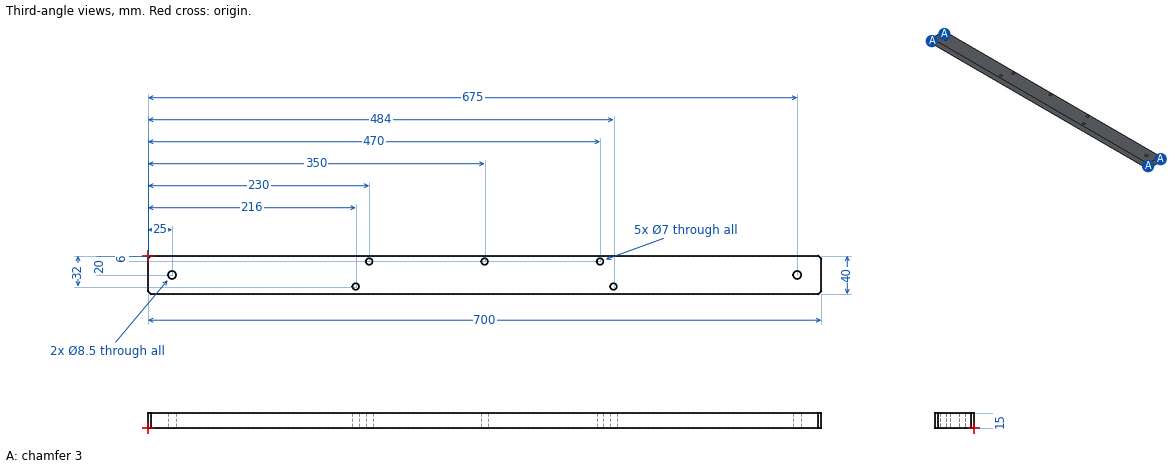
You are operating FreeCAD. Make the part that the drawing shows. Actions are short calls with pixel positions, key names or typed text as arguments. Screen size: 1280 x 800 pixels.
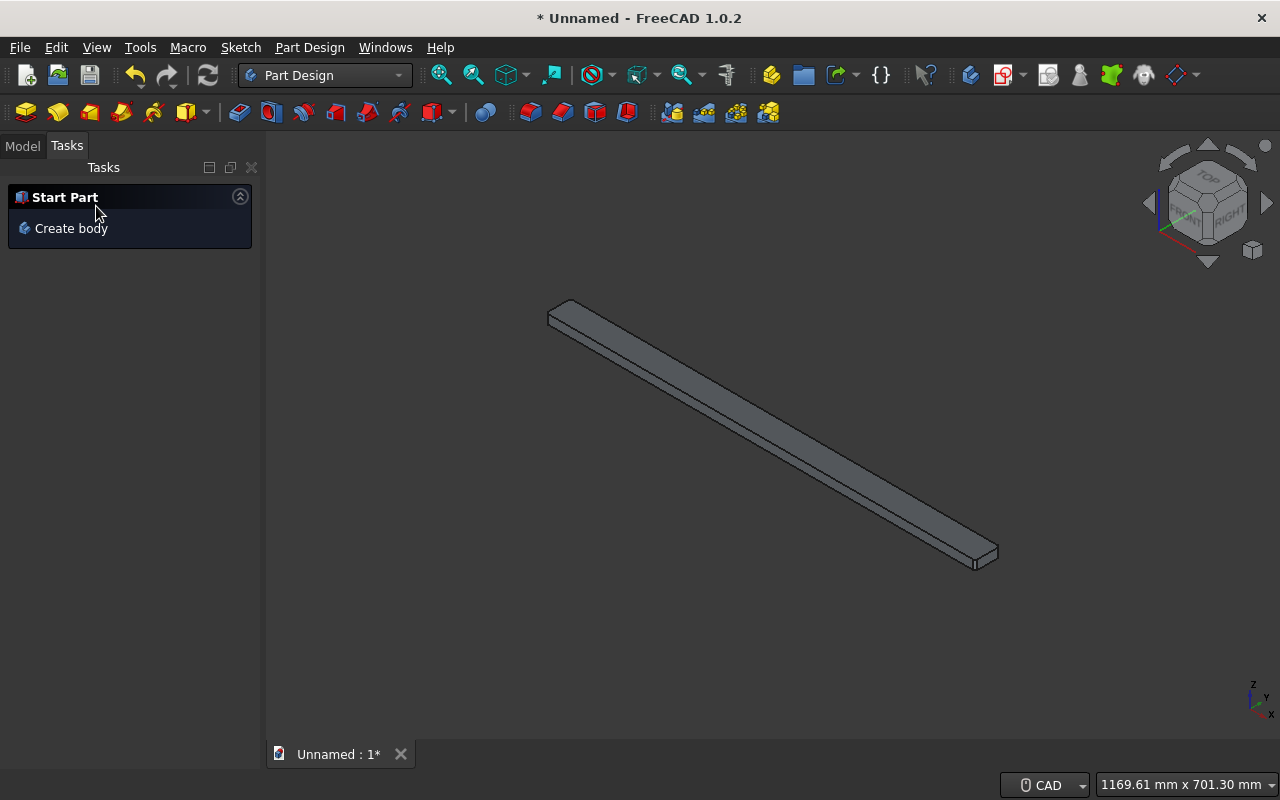
click(442, 76)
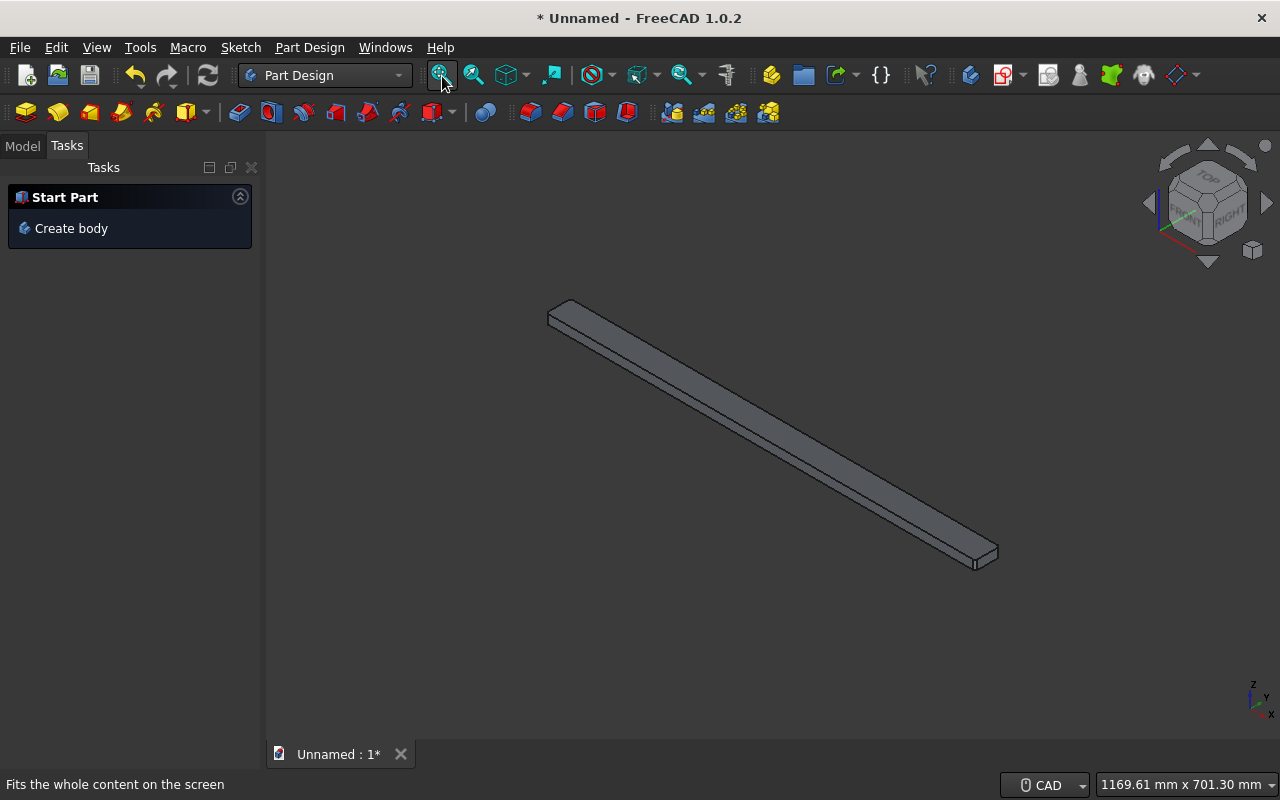
click(957, 535)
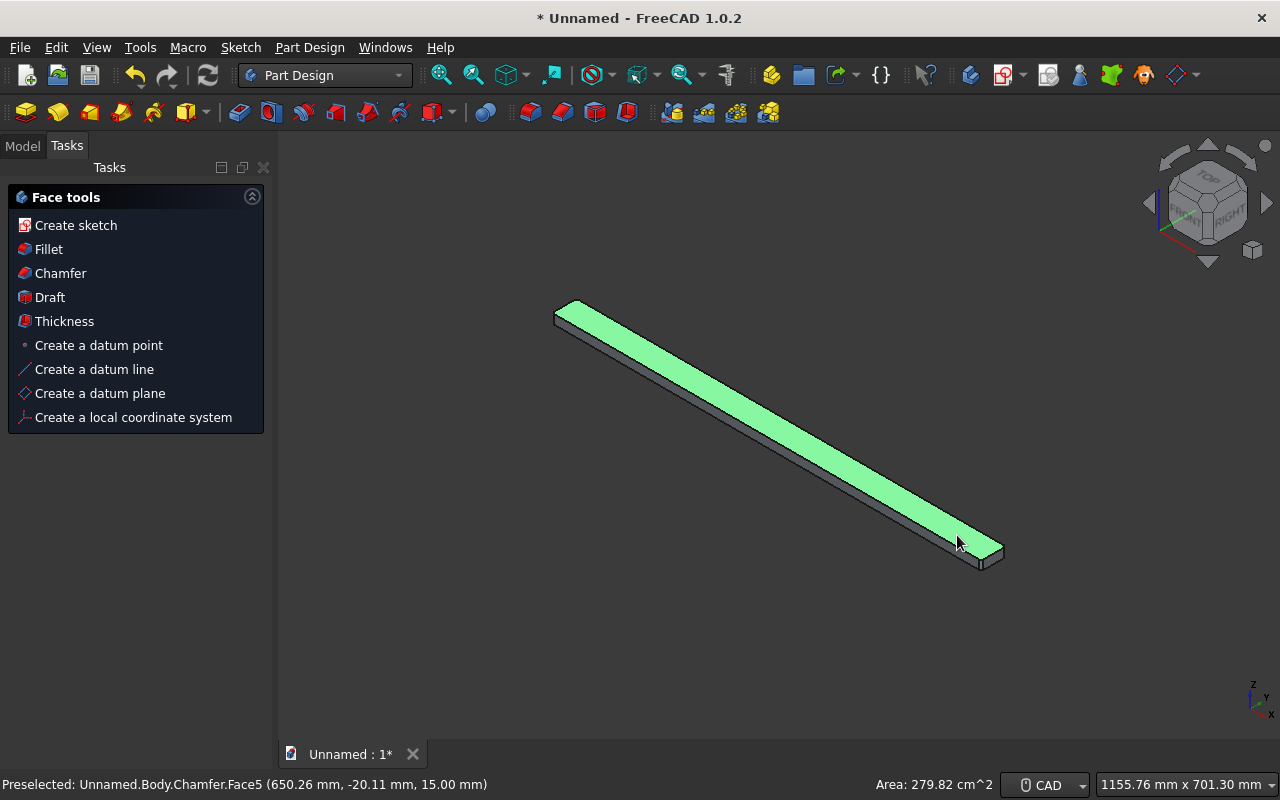
click(1004, 76)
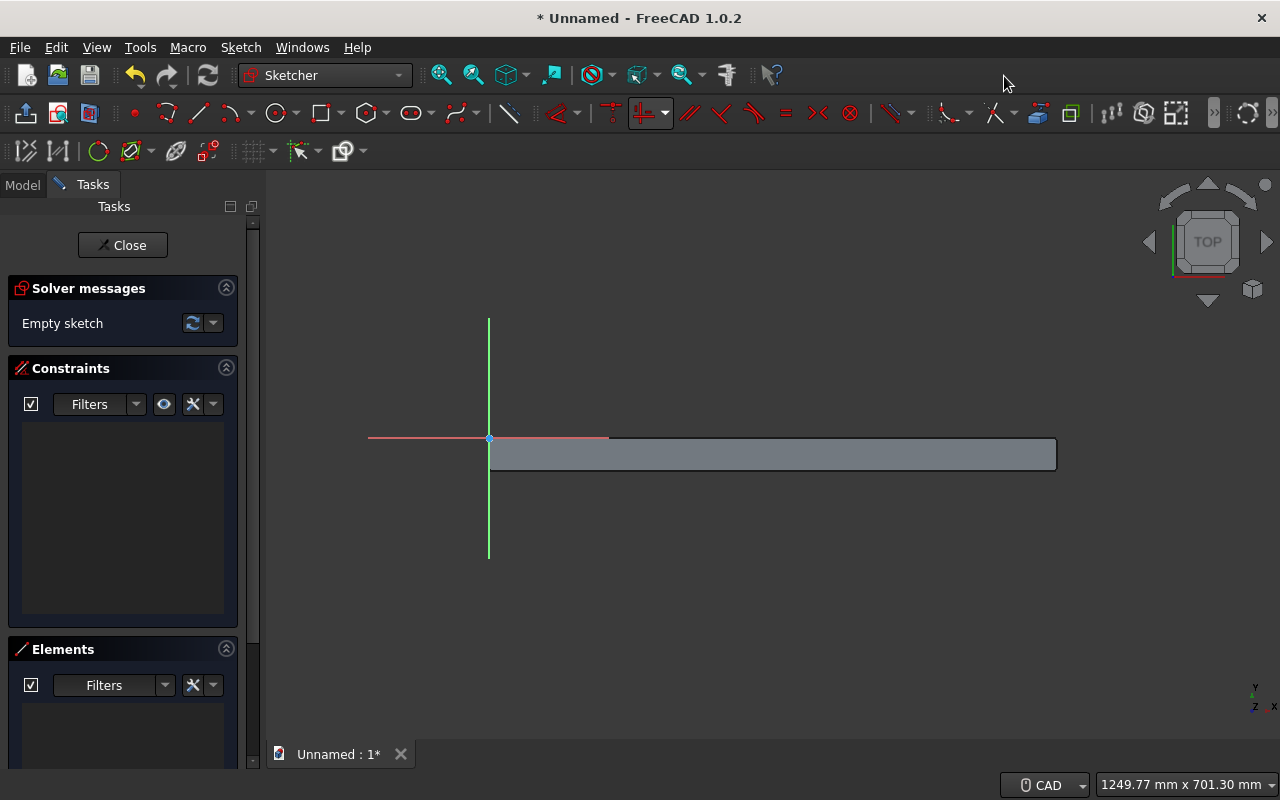
click(276, 114)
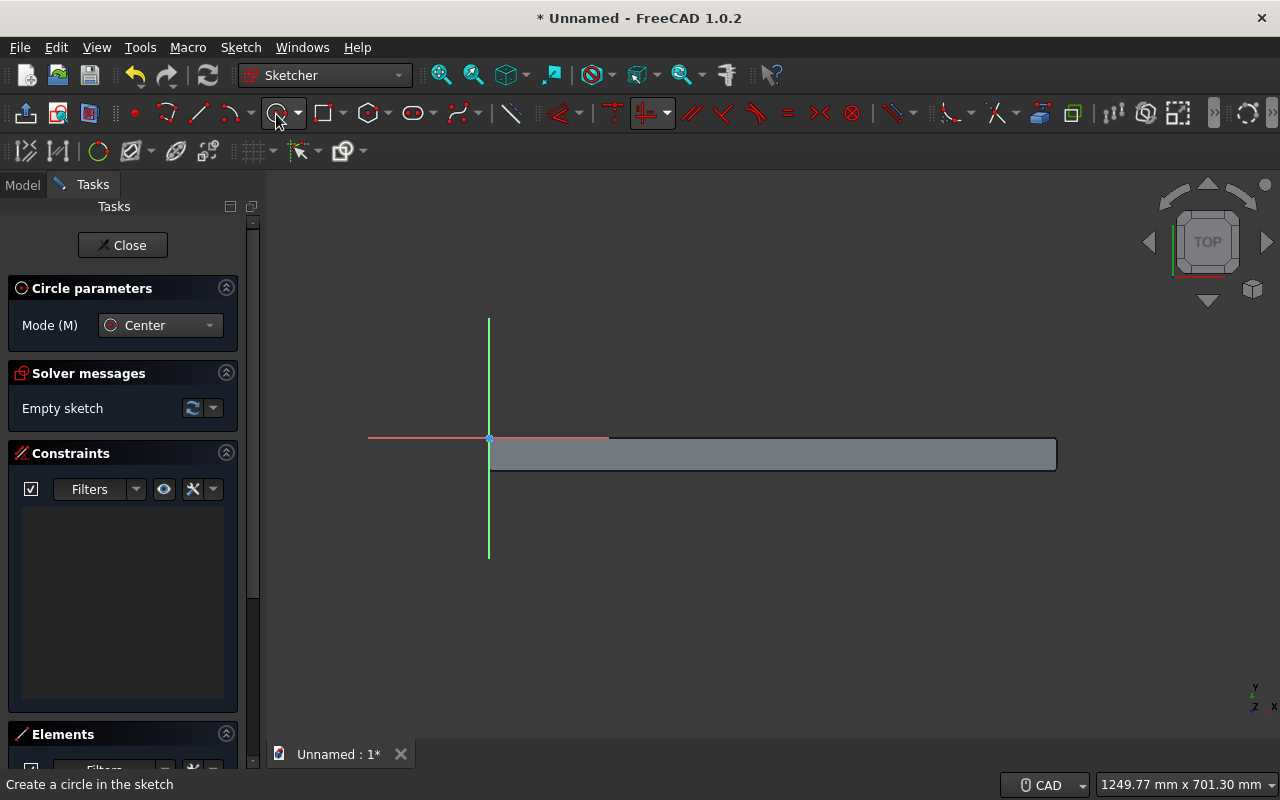
scroll(509, 454, up, 10)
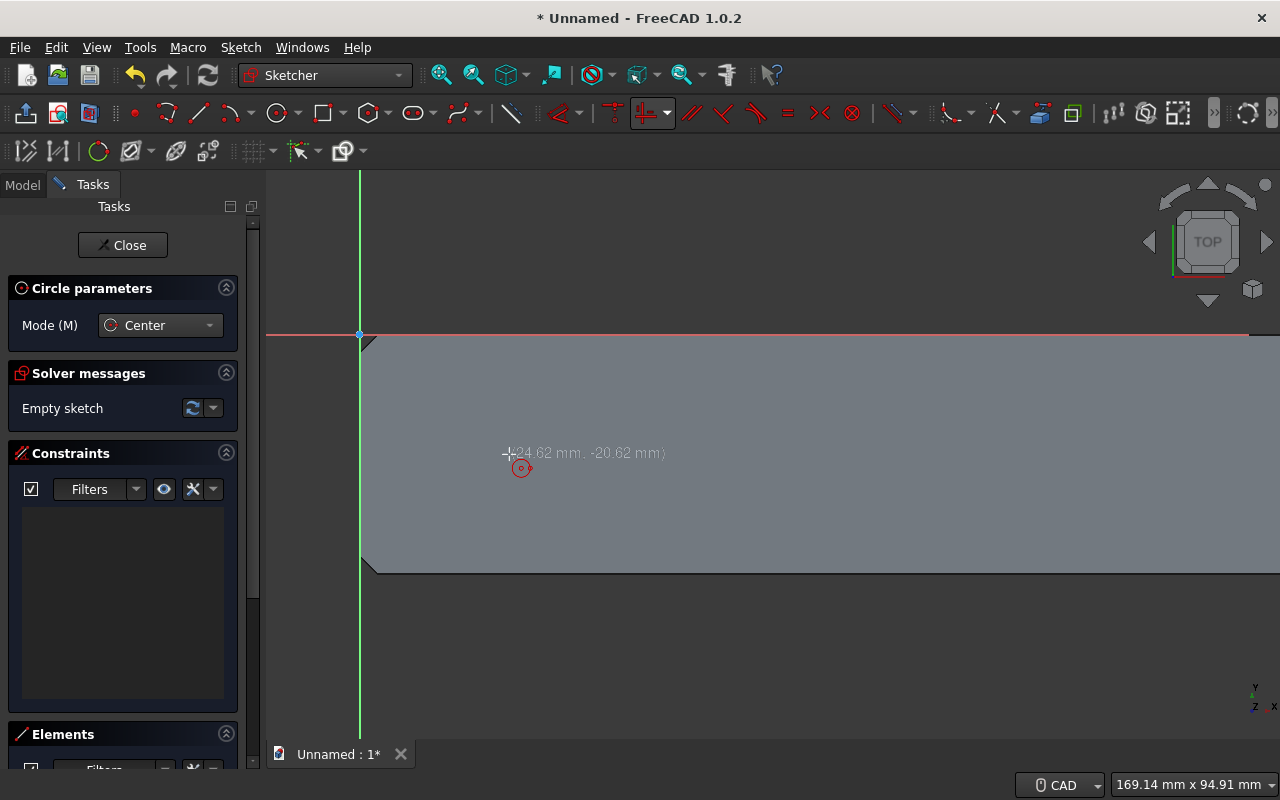
scroll(440, 462, down, 10)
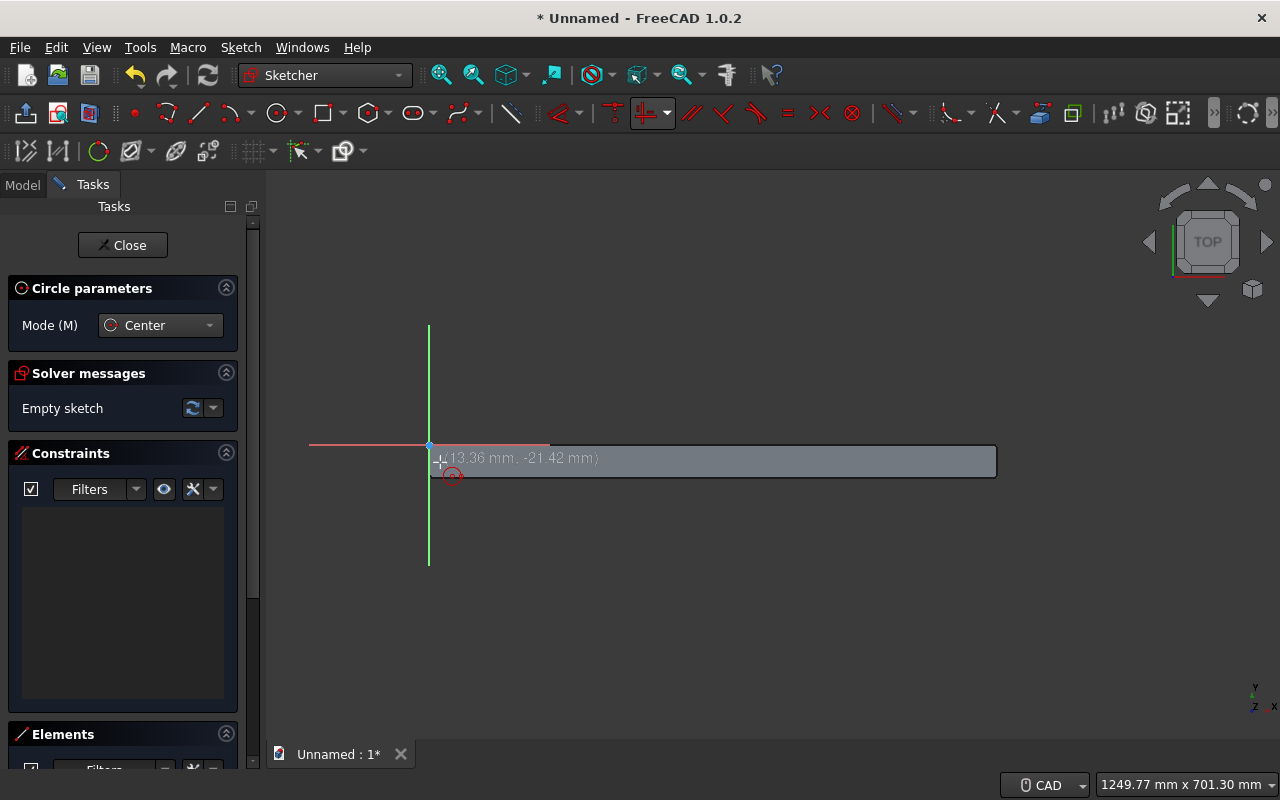
click(450, 461)
move(452, 464)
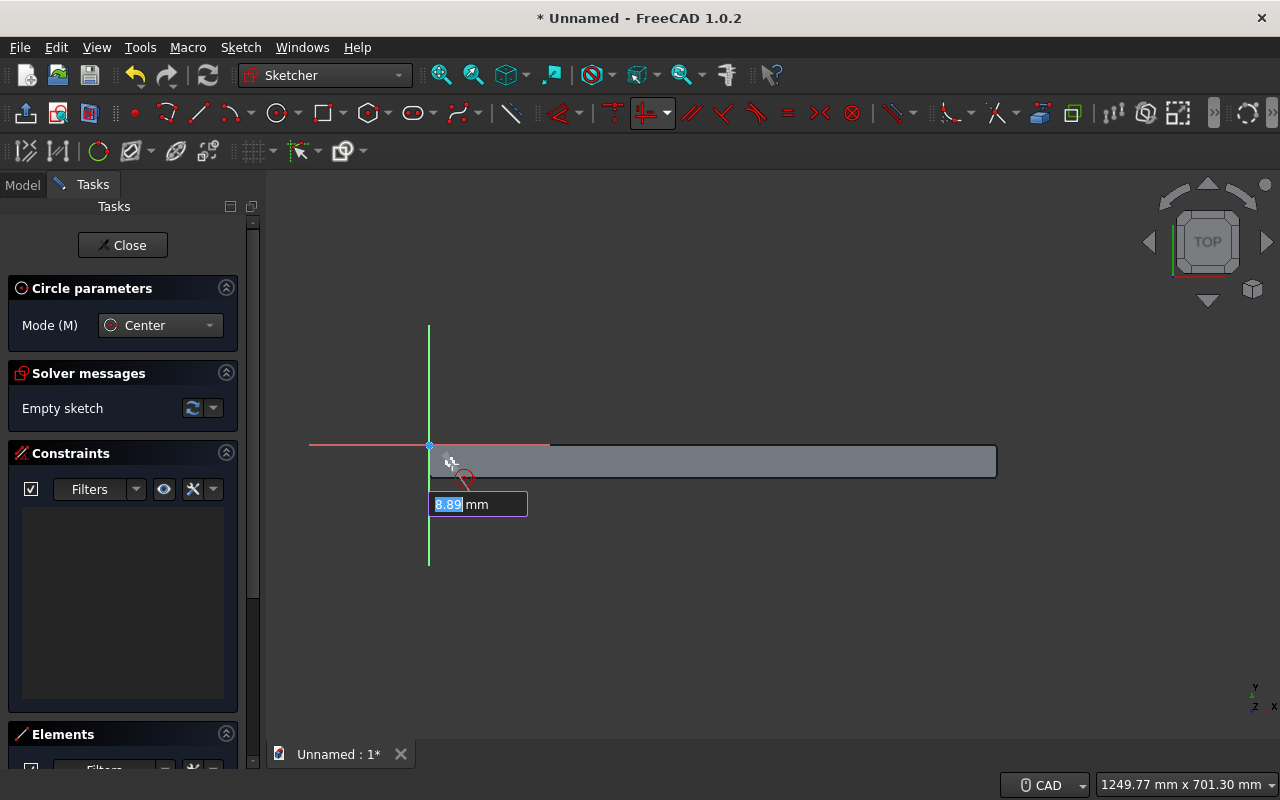
text(8.5)
key(Return)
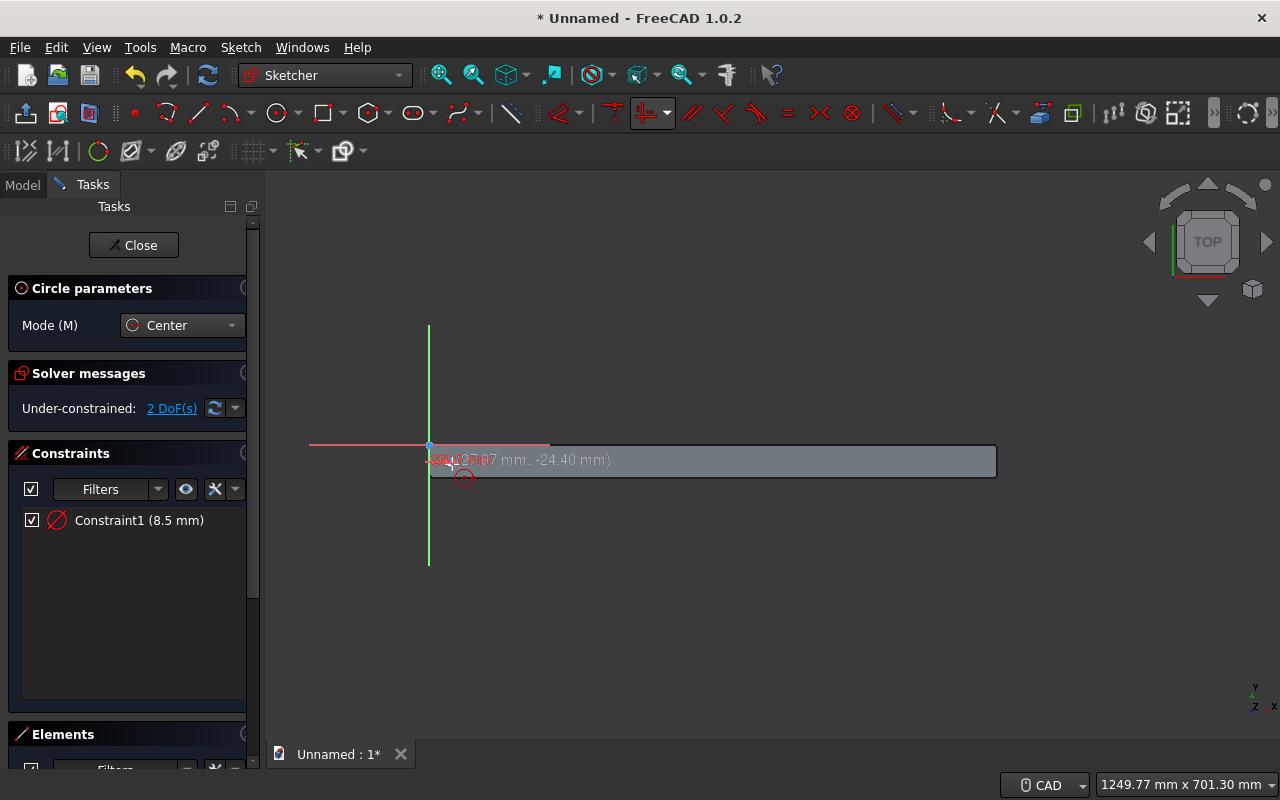
scroll(977, 461, up, 10)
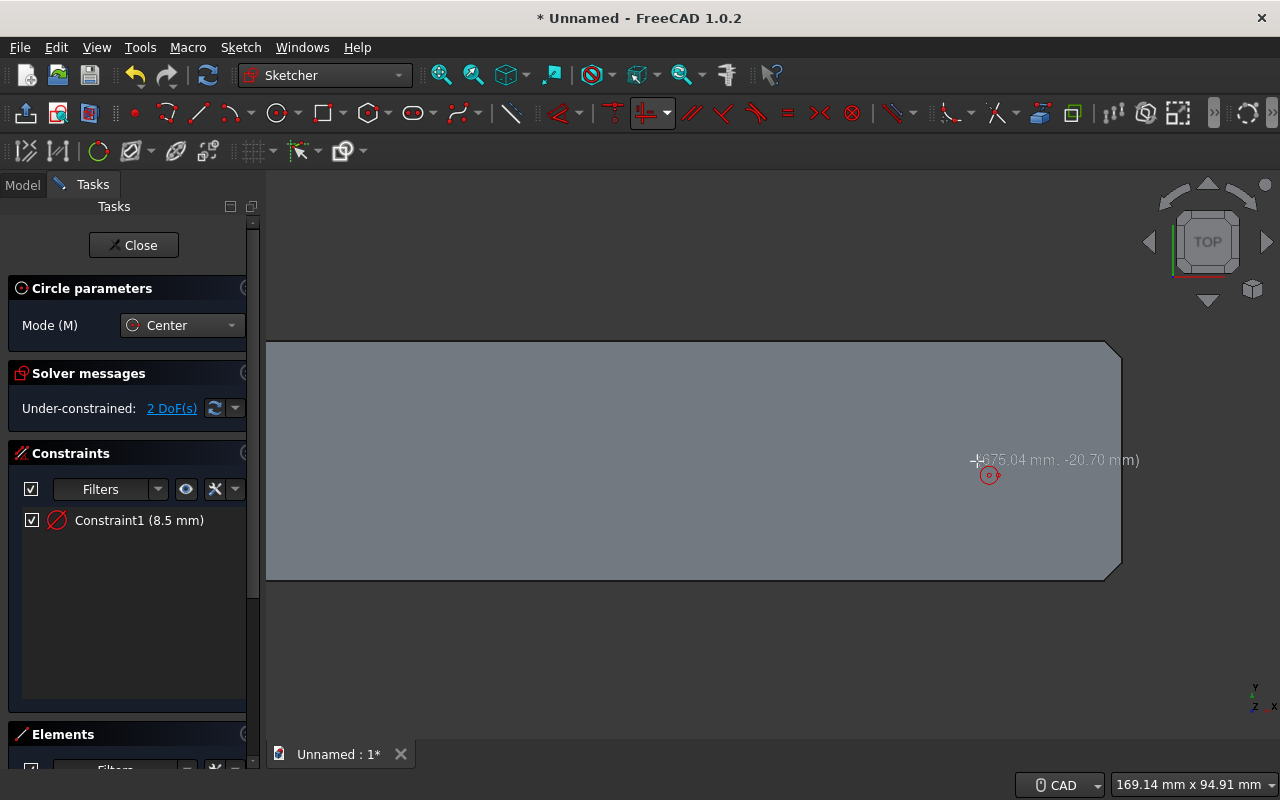
scroll(977, 461, down, 10)